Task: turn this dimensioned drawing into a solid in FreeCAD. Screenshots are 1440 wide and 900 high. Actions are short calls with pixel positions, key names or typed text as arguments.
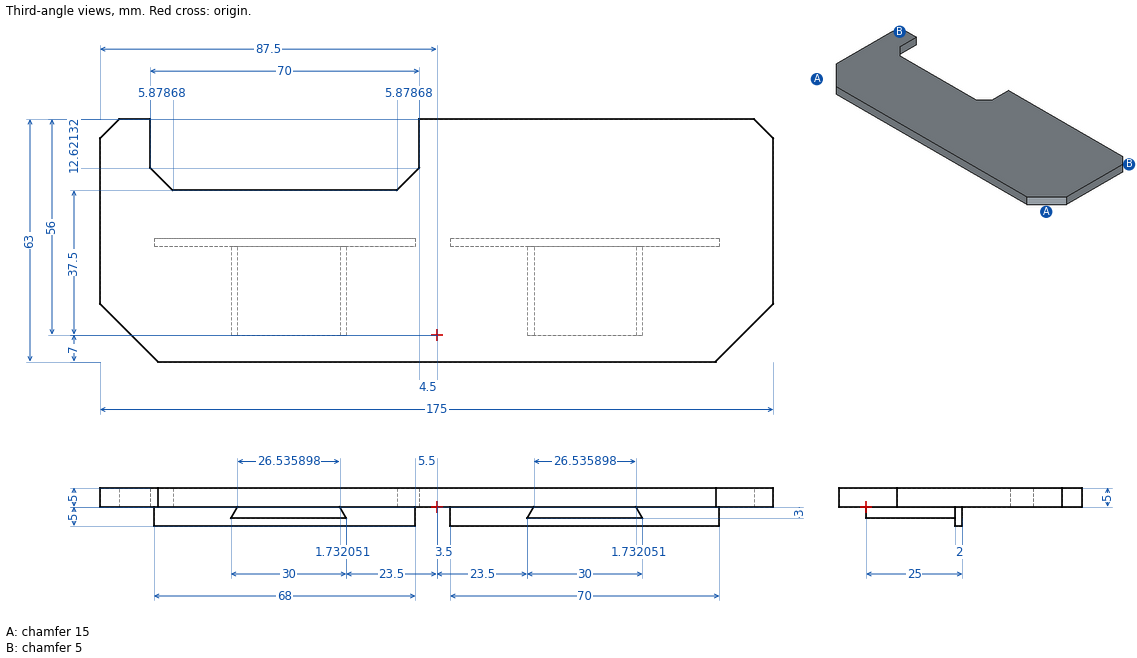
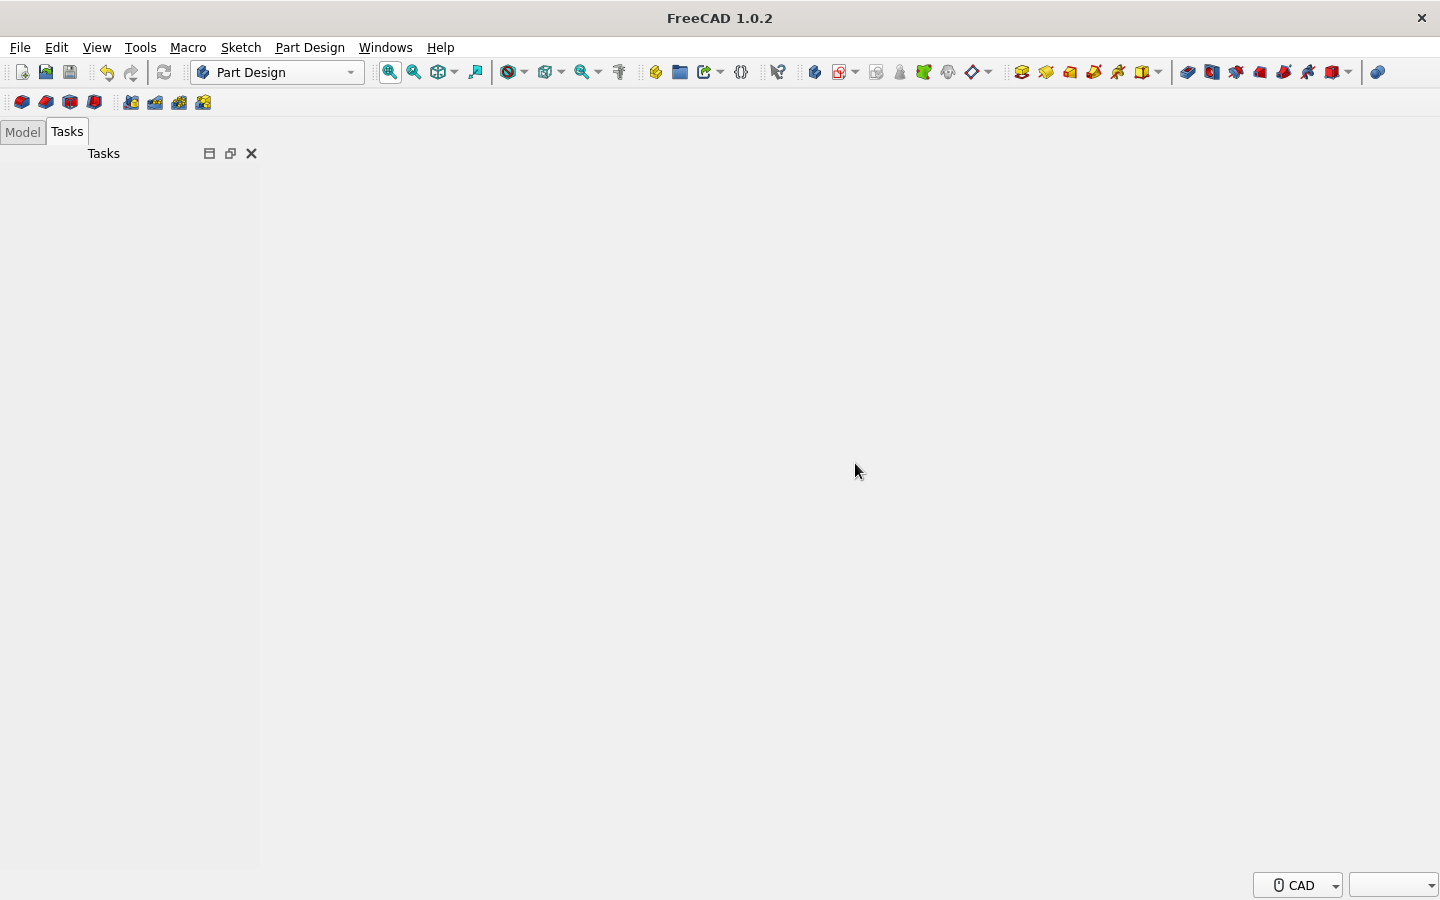
key(ctrl+n)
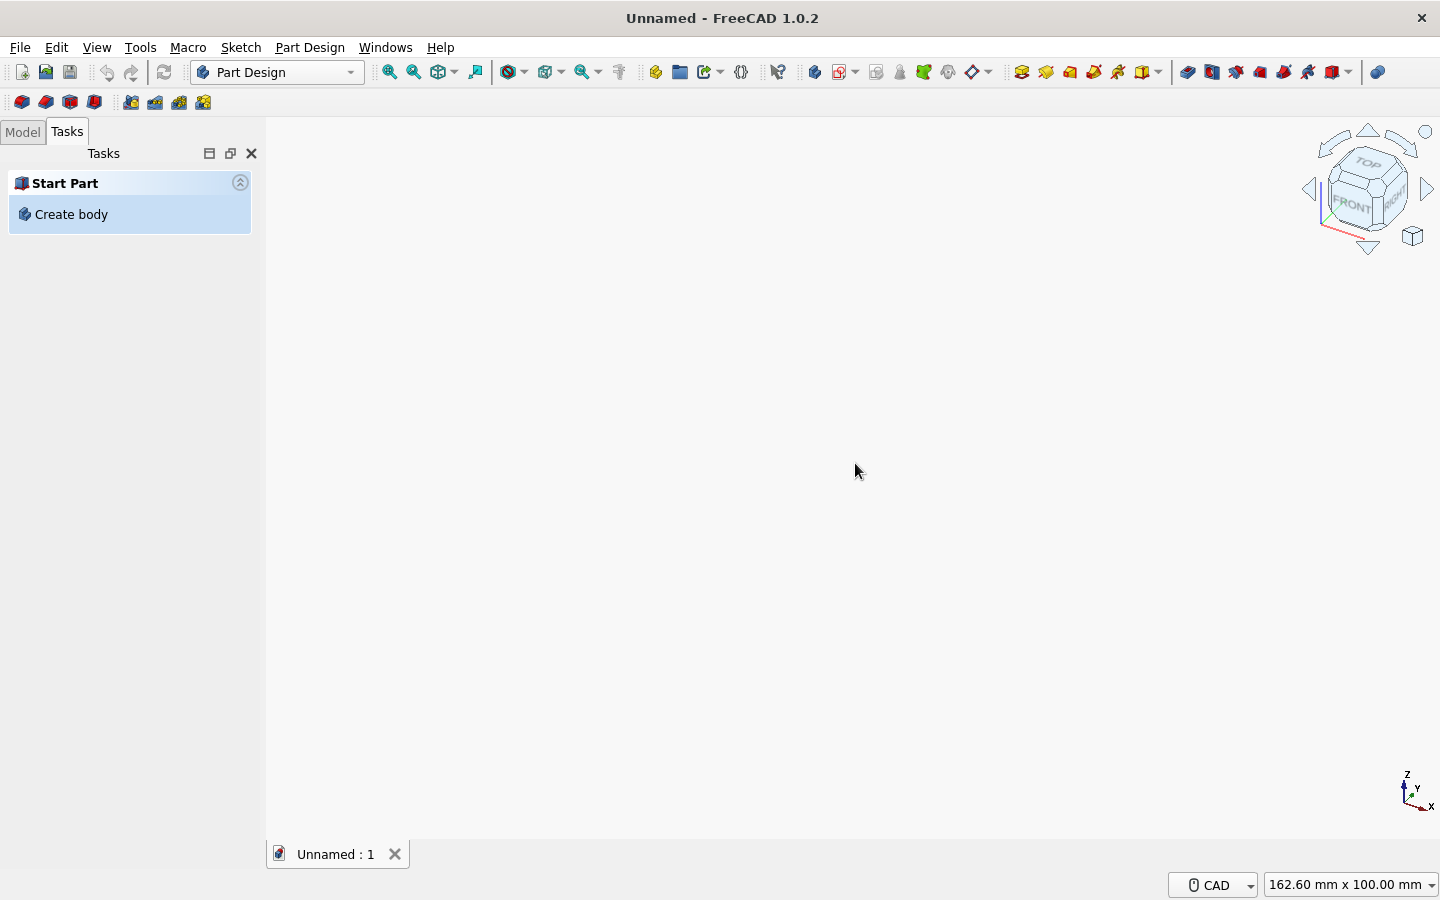
click(840, 72)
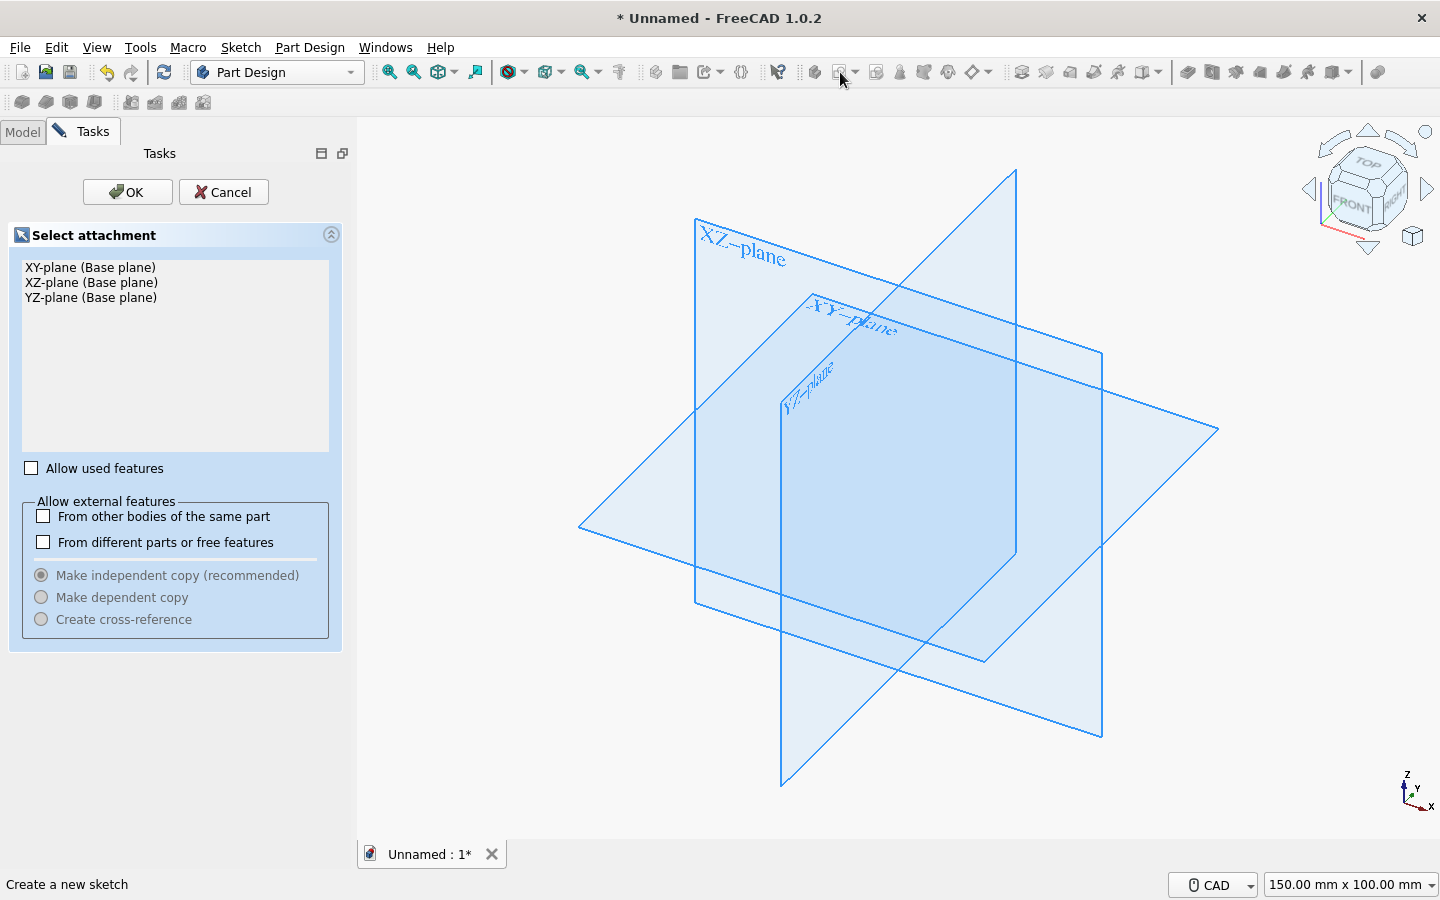
click(82, 268)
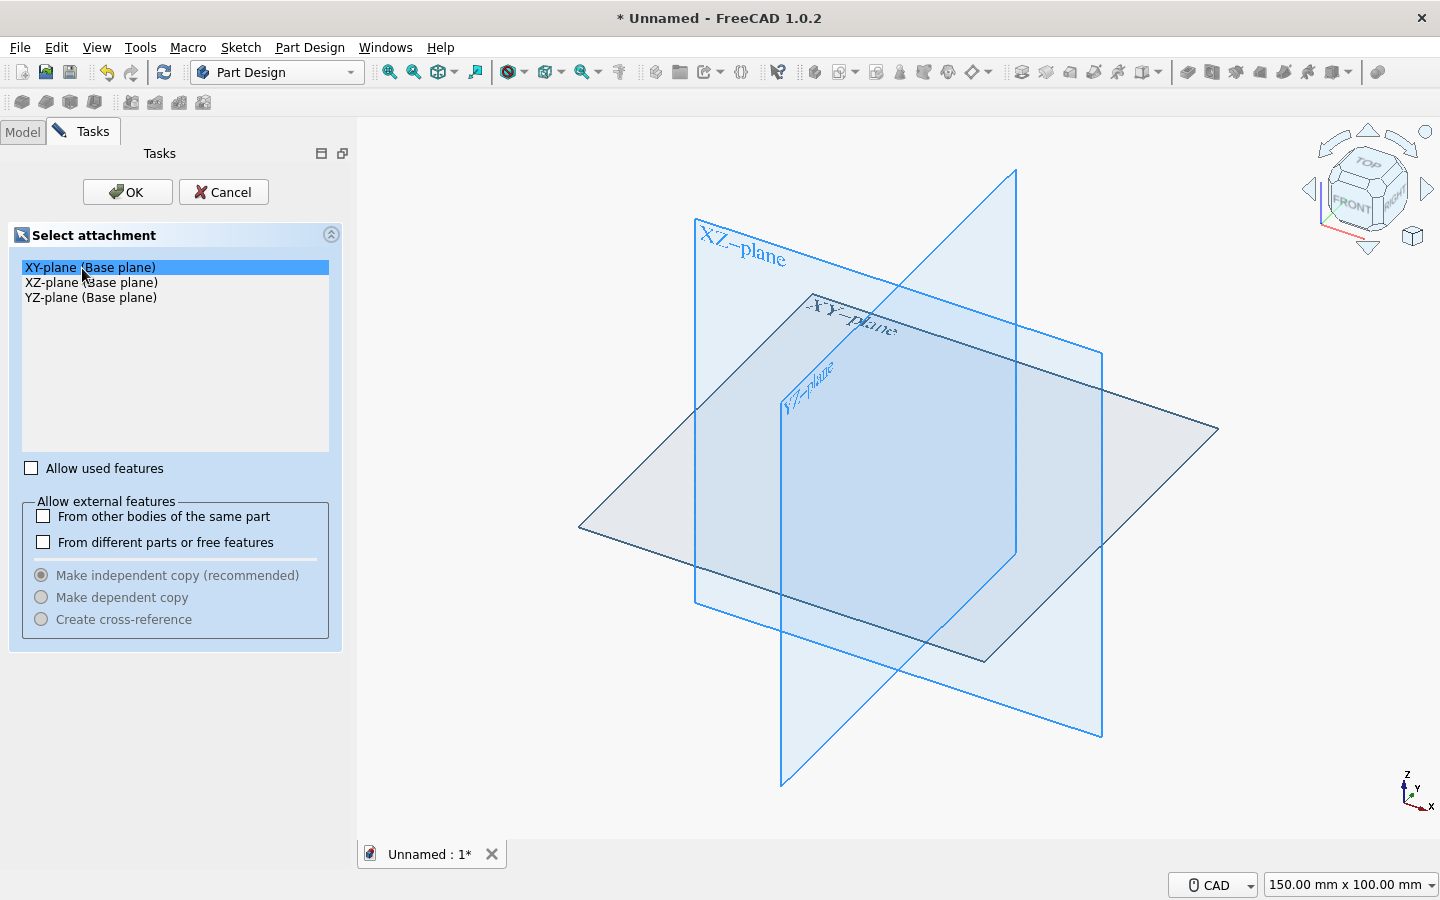
click(128, 192)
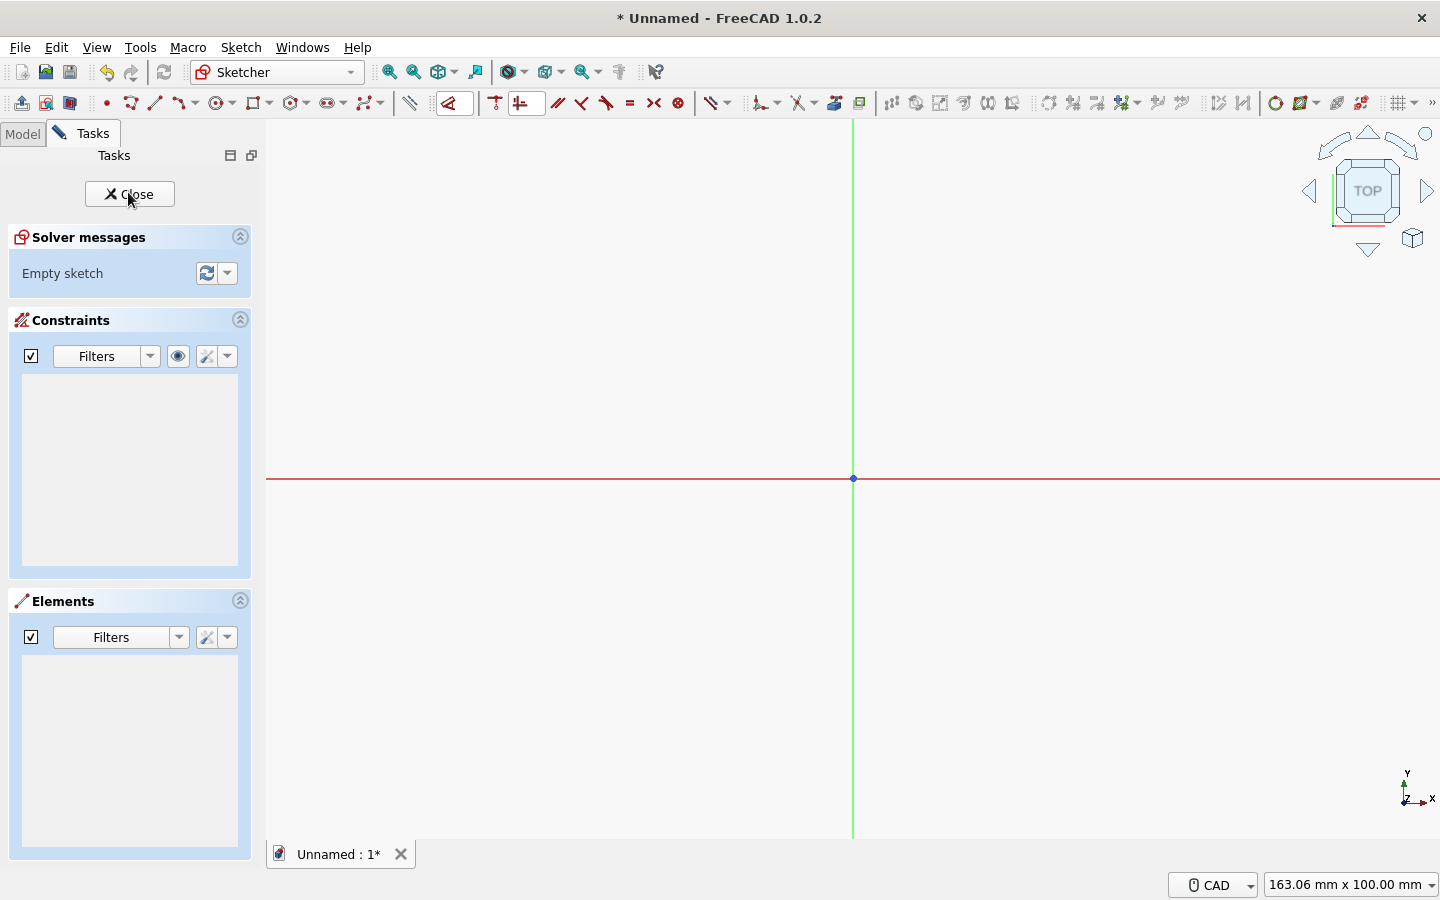
scroll(701, 694, down, 3)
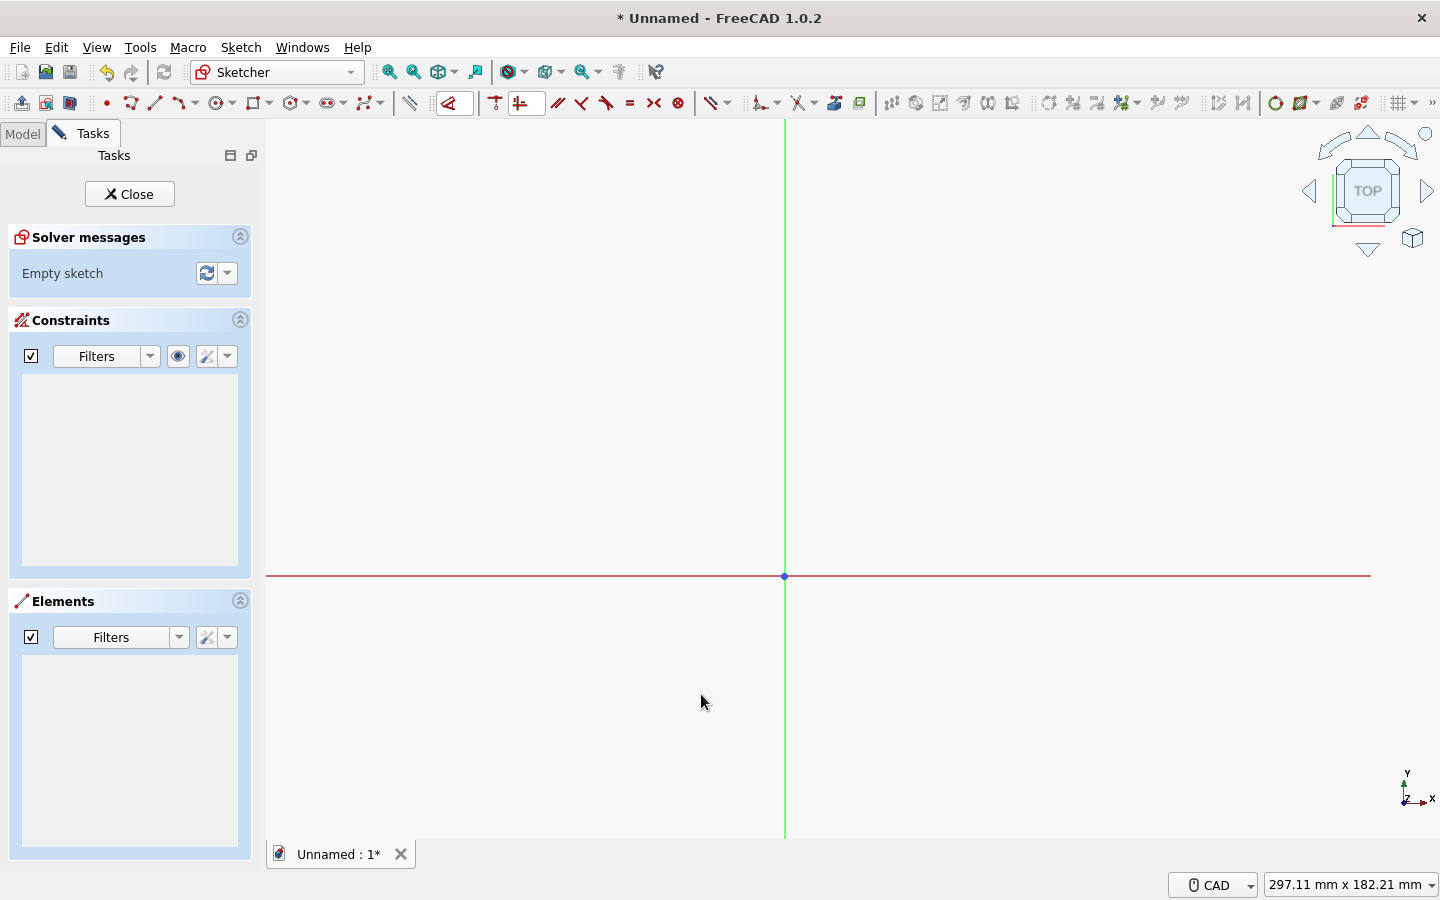
click(254, 104)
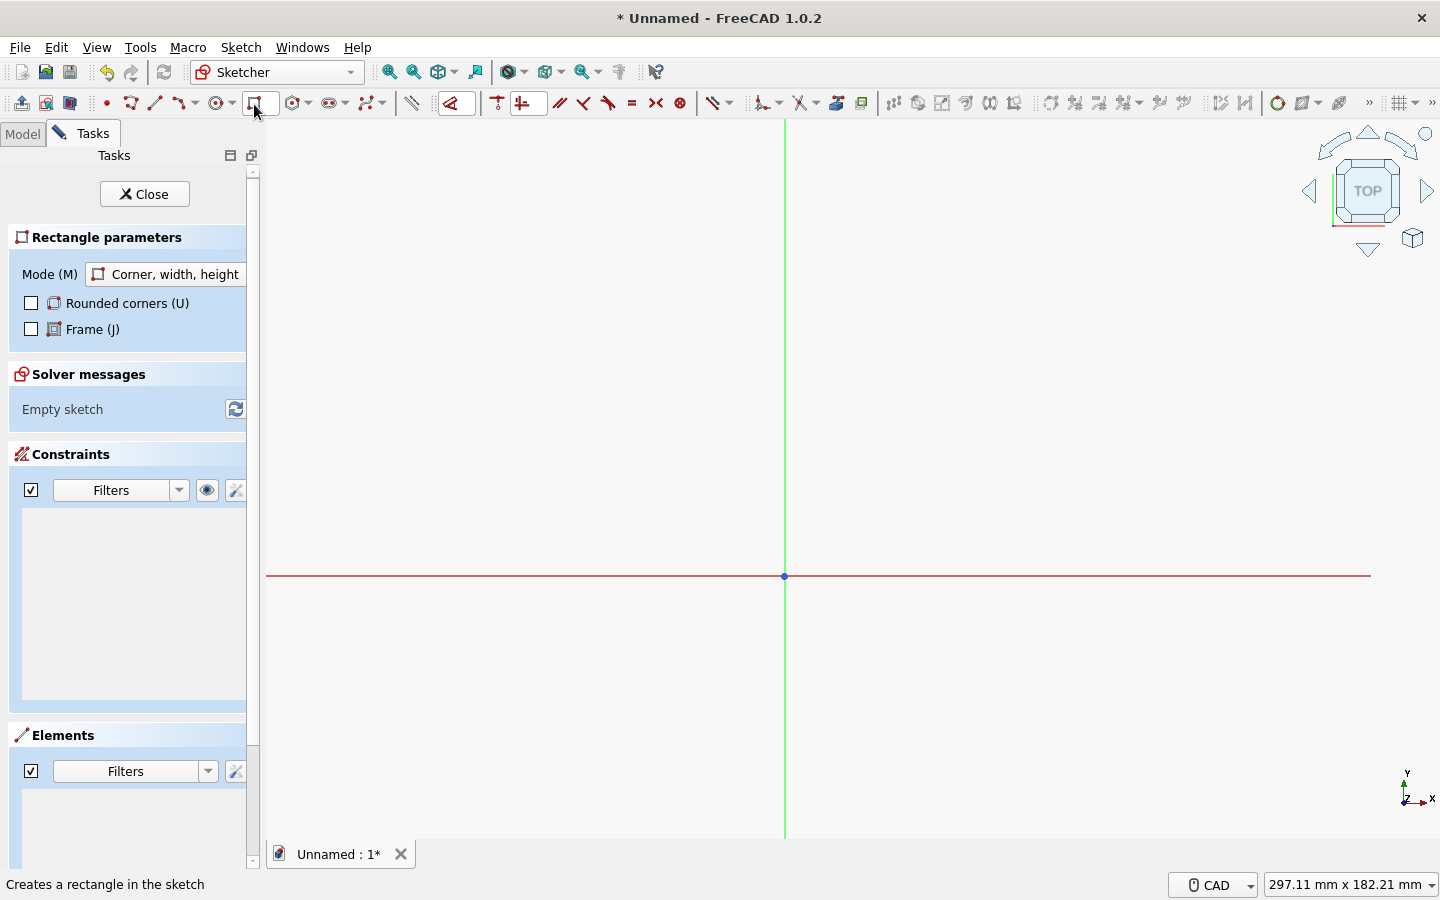
click(439, 355)
click(1130, 604)
key(Escape)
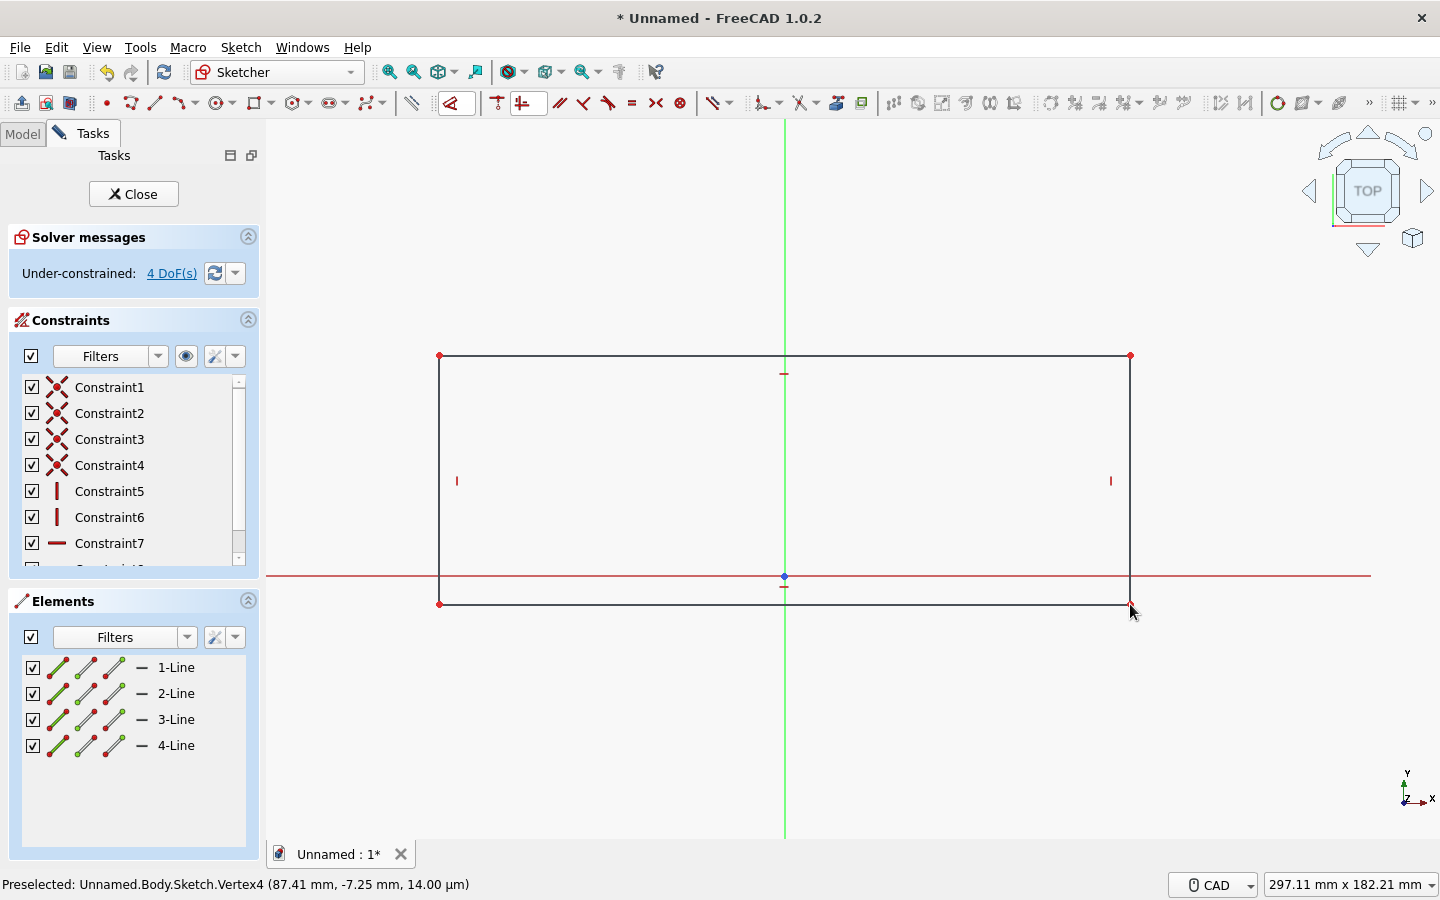
click(439, 431)